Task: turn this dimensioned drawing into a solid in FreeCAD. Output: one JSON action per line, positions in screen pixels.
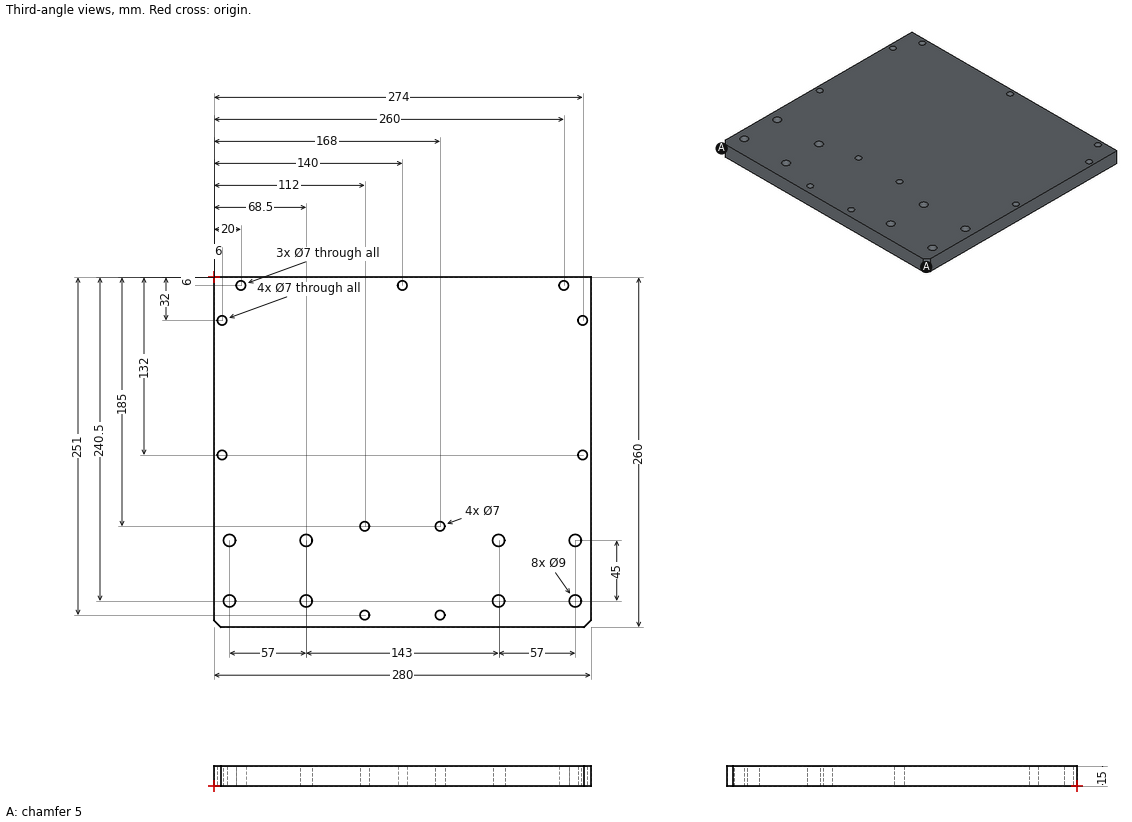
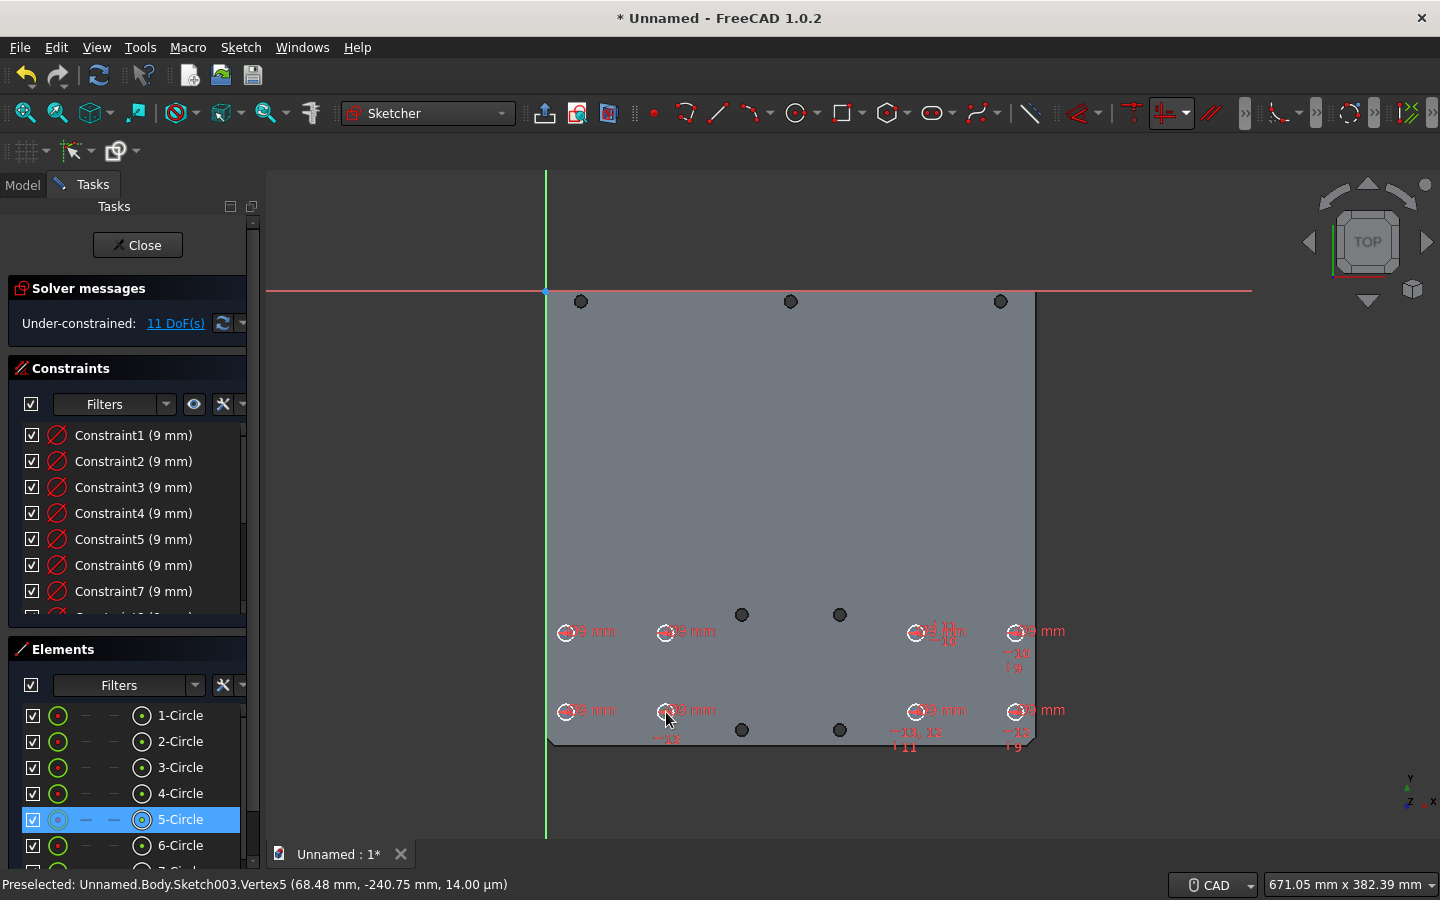
{"action": "left_click", "coordinate": [666, 633]}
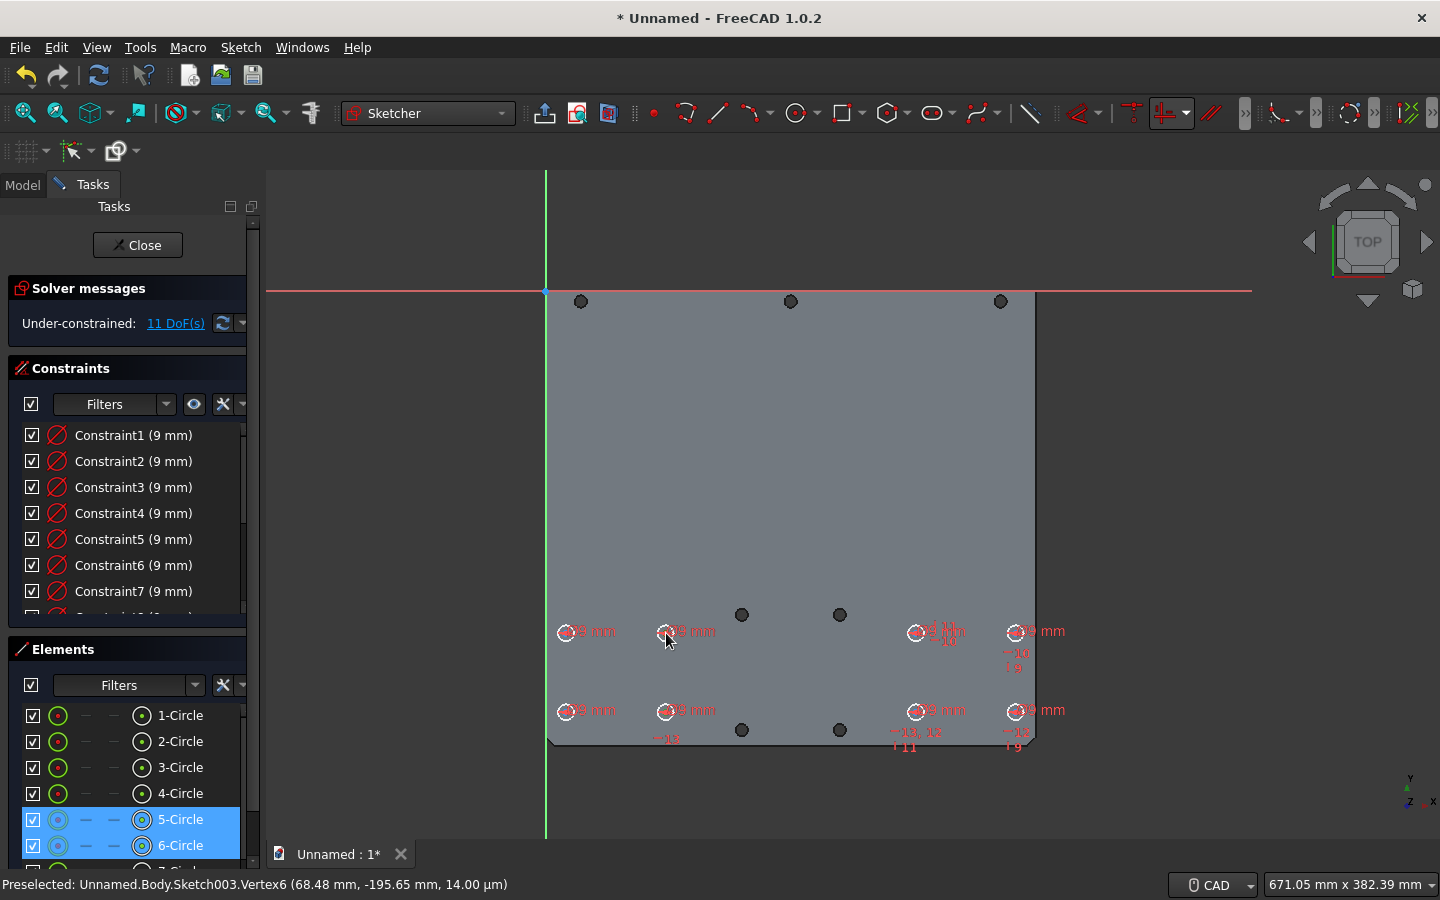
{"action": "left_click", "coordinate": [1188, 114]}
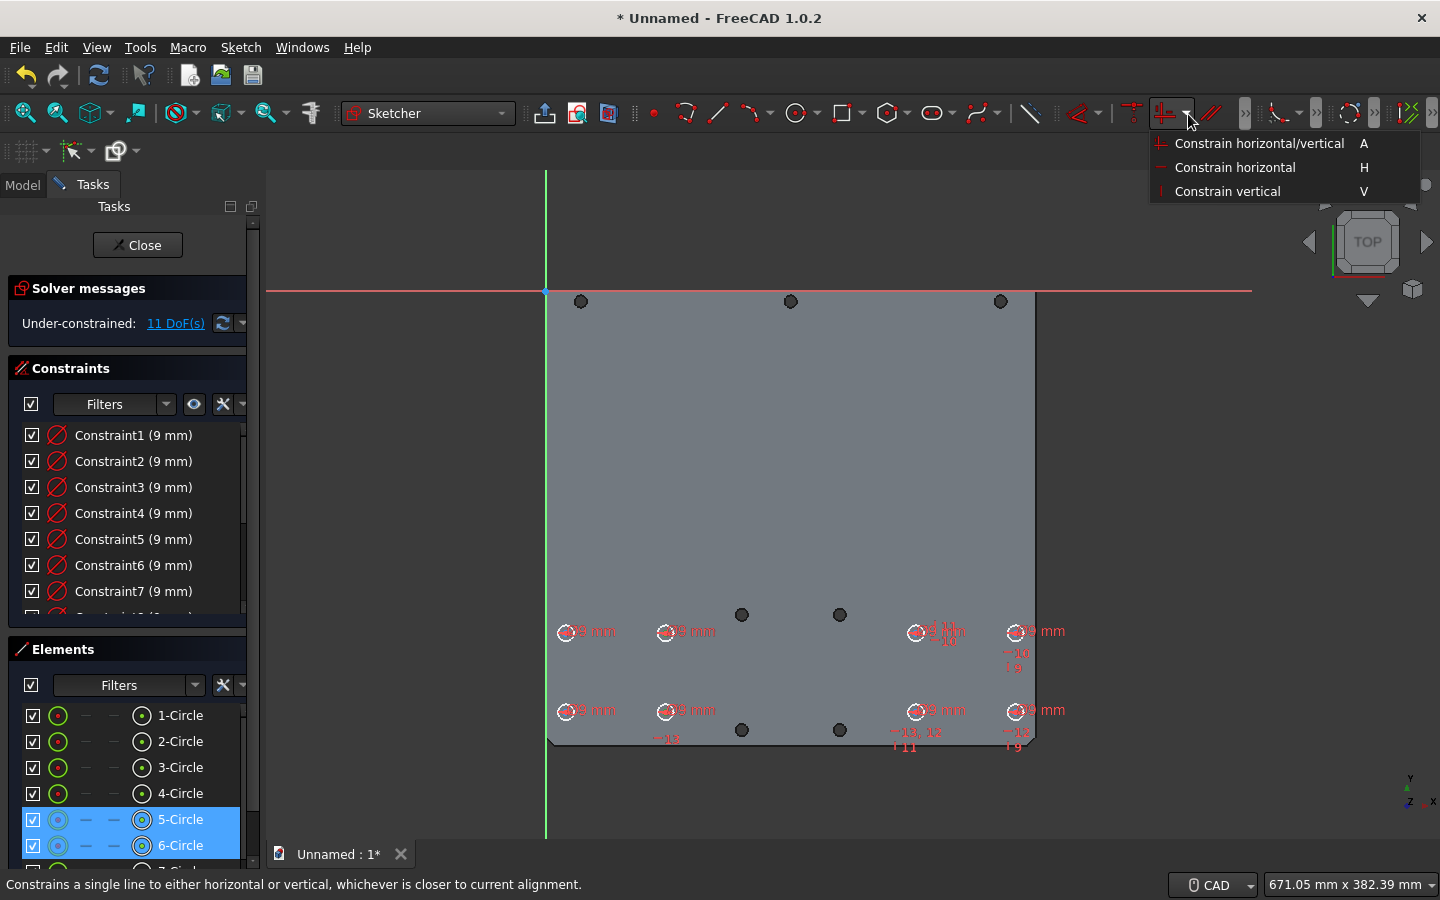
{"action": "left_click", "coordinate": [1285, 191]}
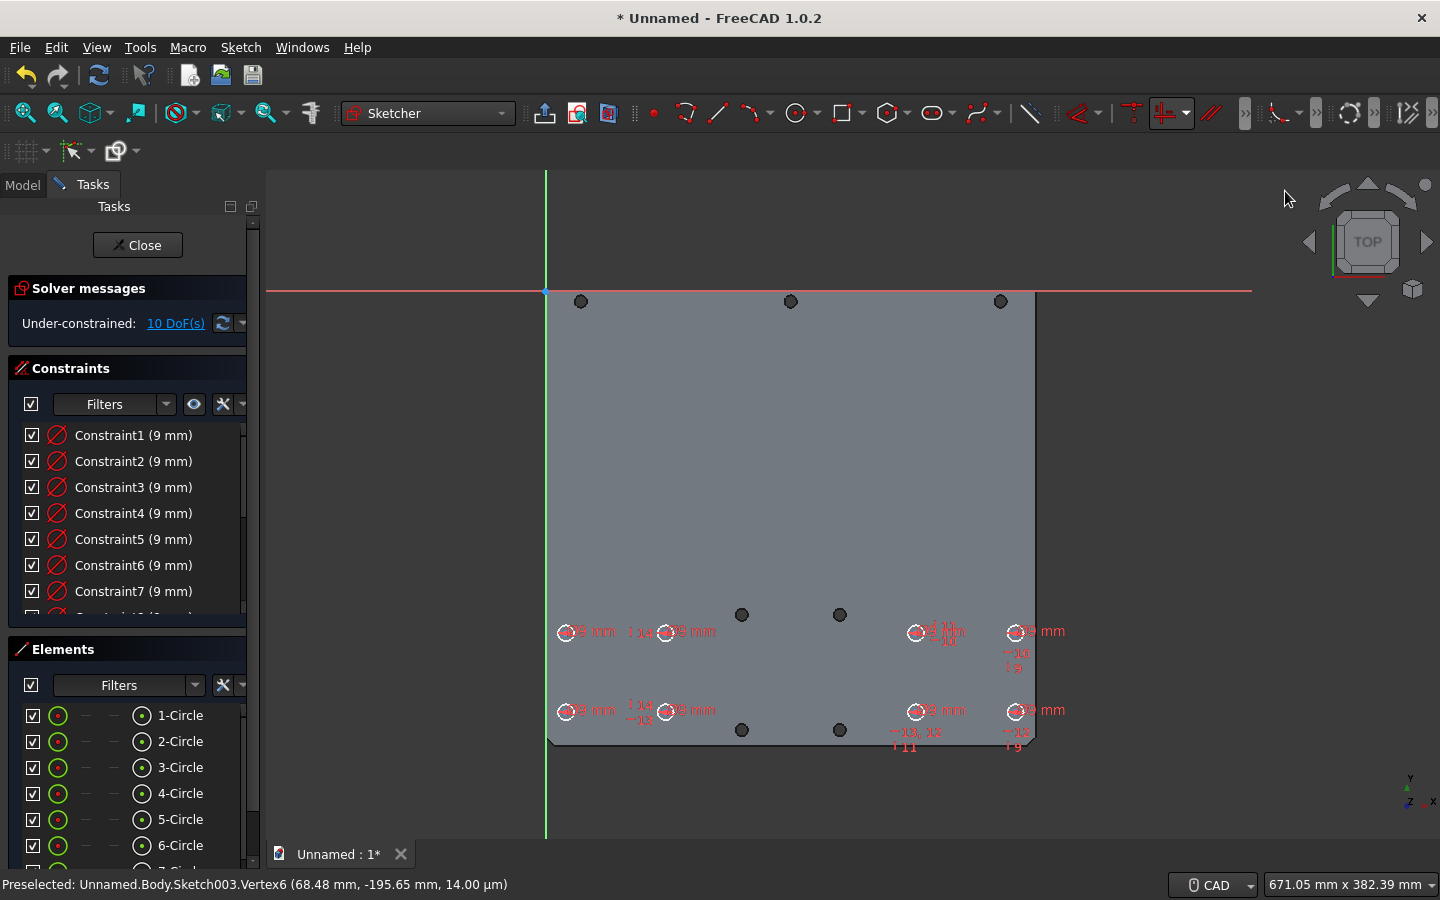
{"action": "left_click", "coordinate": [916, 633]}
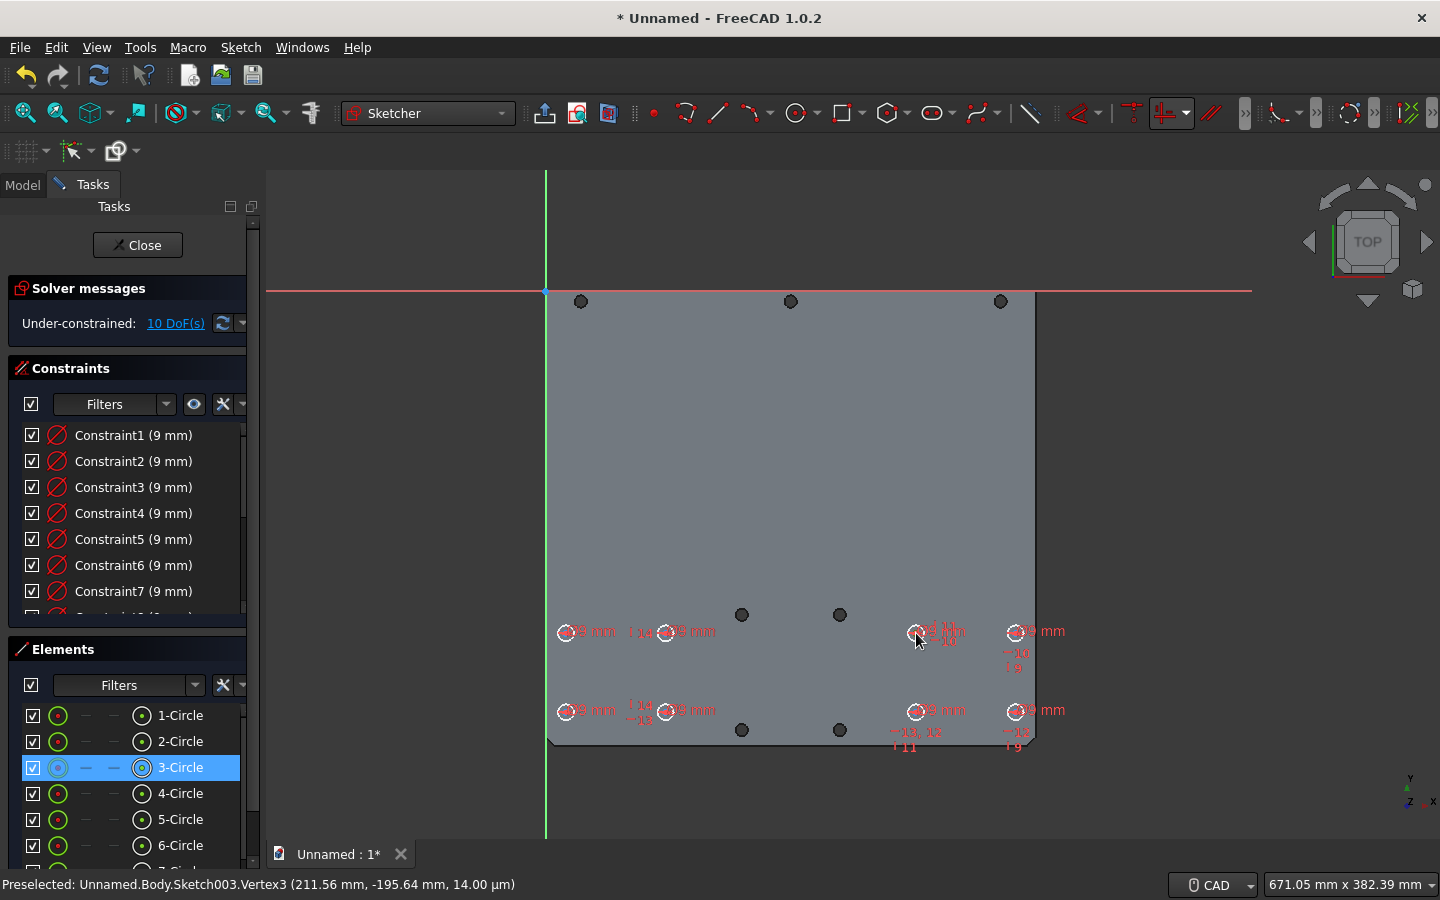
{"action": "left_click", "coordinate": [666, 633]}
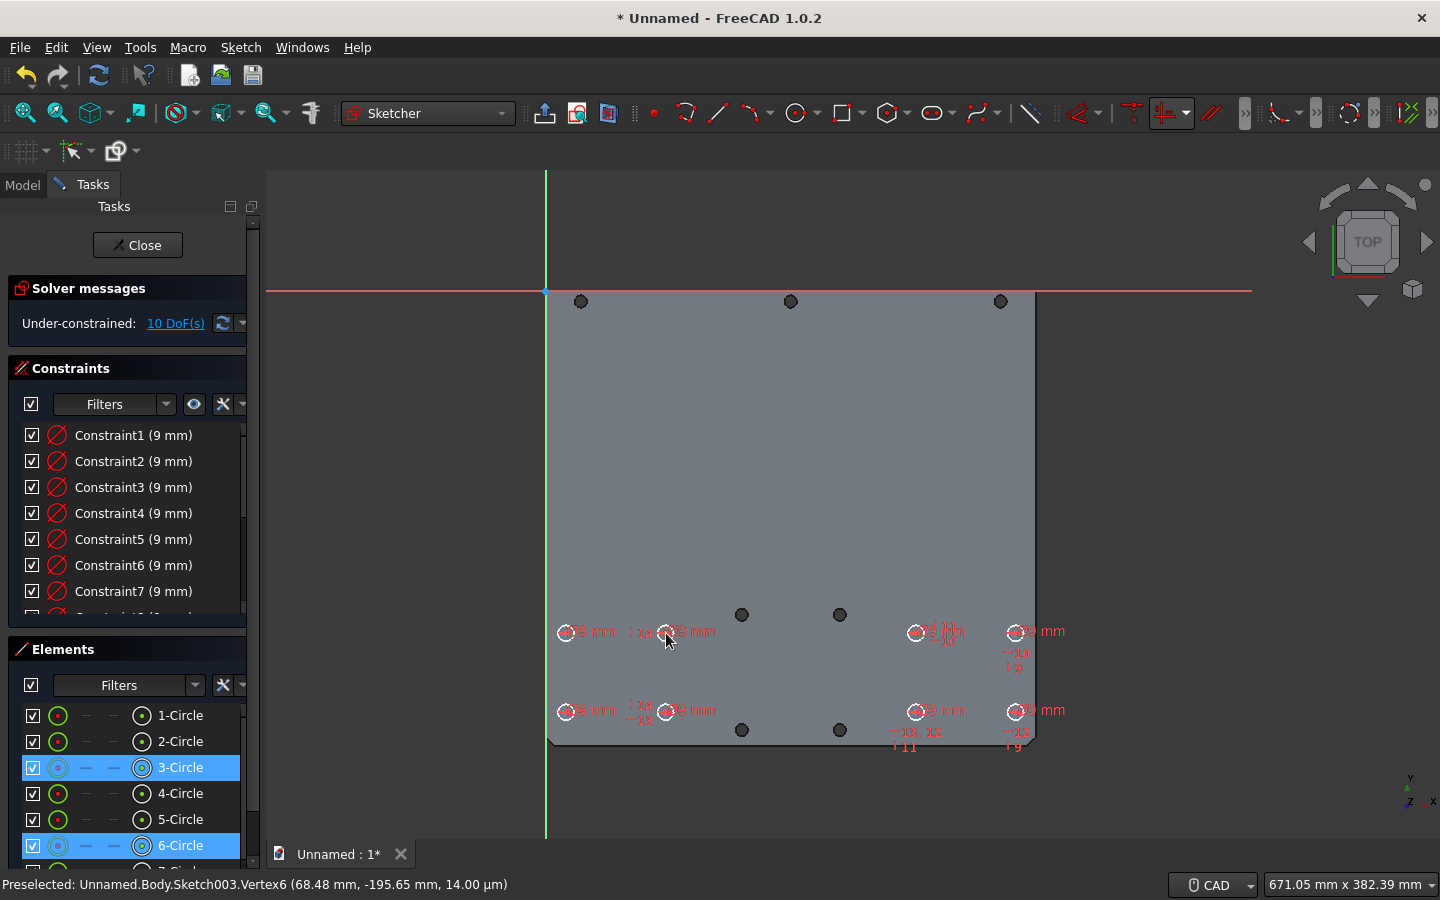
{"action": "left_click", "coordinate": [1188, 114]}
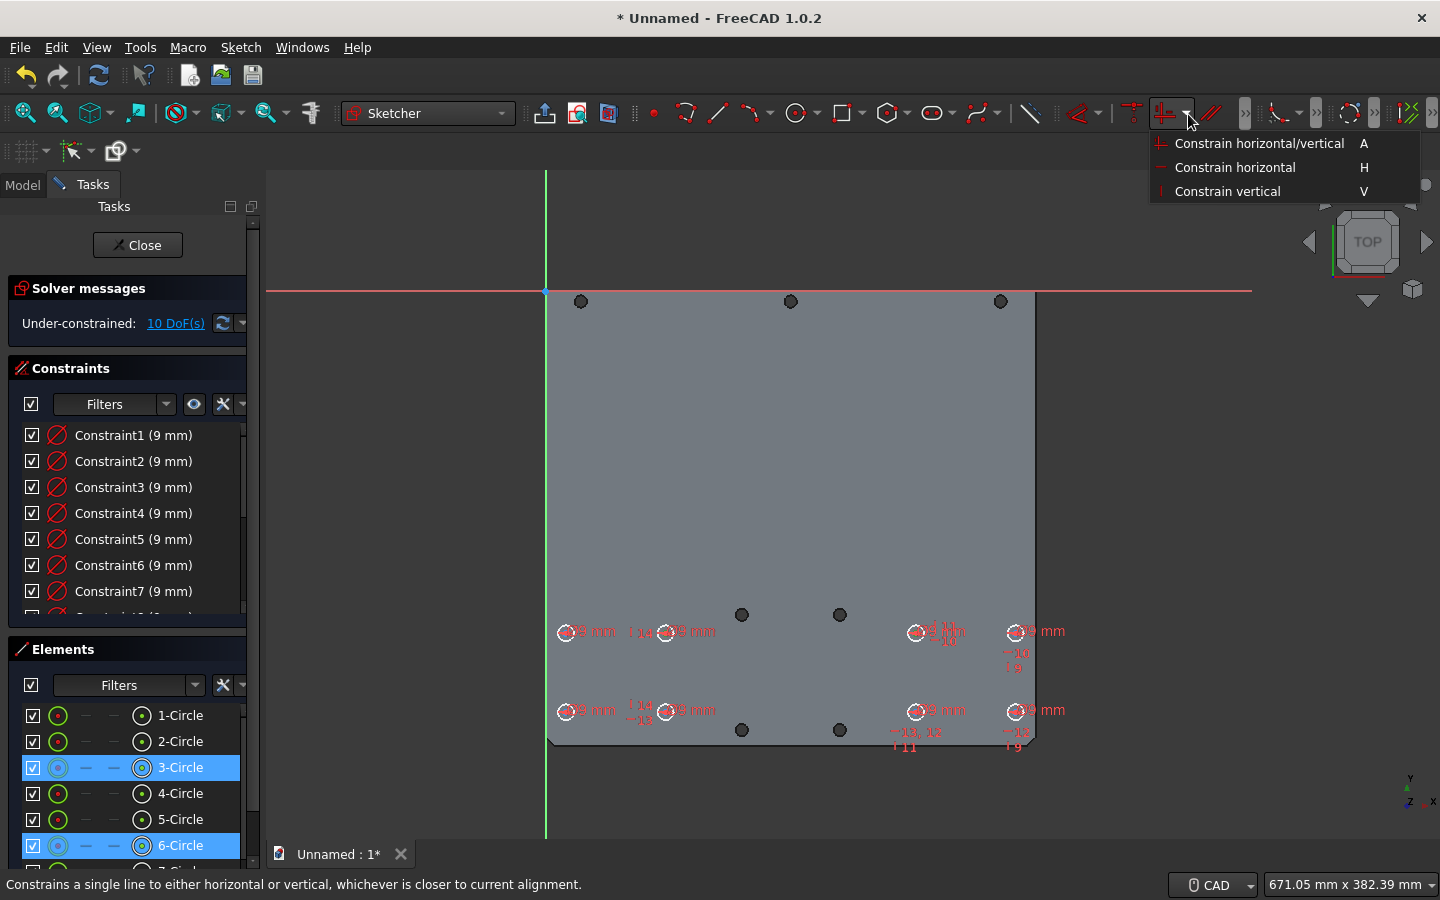
{"action": "left_click", "coordinate": [1285, 167]}